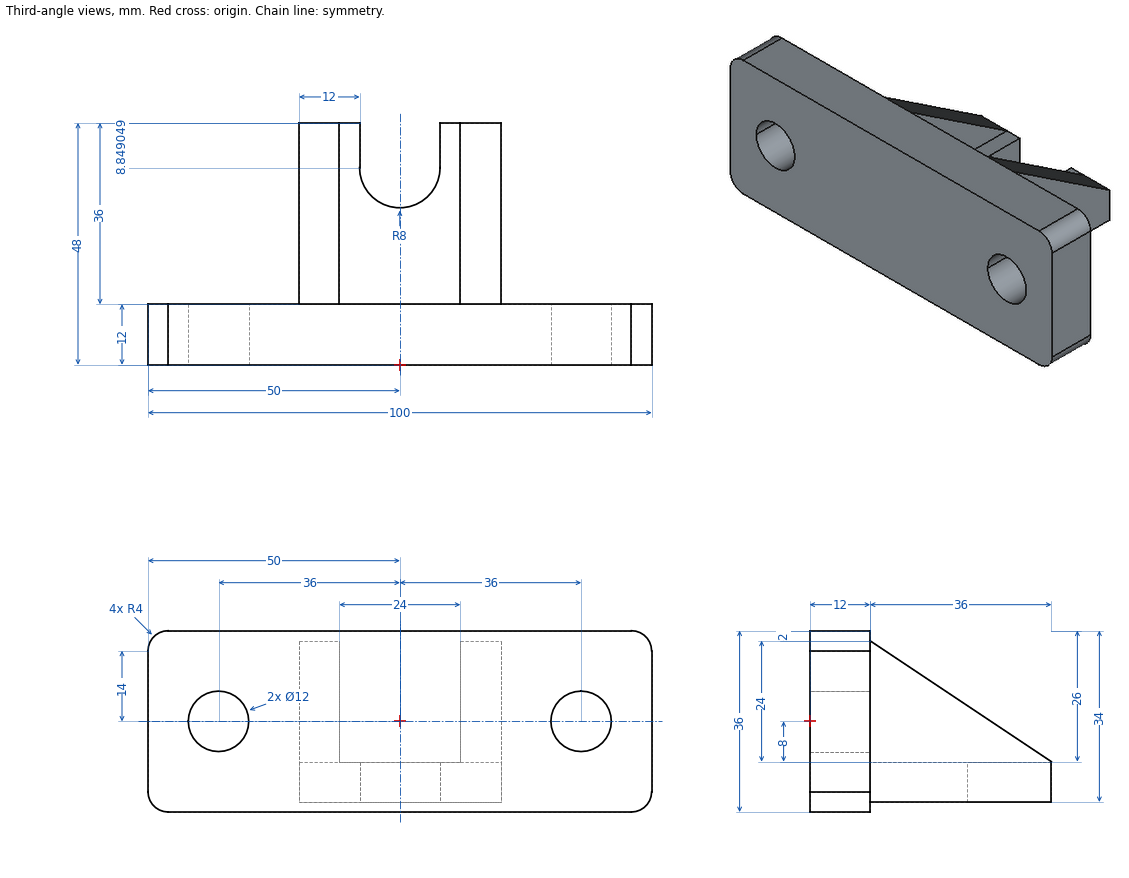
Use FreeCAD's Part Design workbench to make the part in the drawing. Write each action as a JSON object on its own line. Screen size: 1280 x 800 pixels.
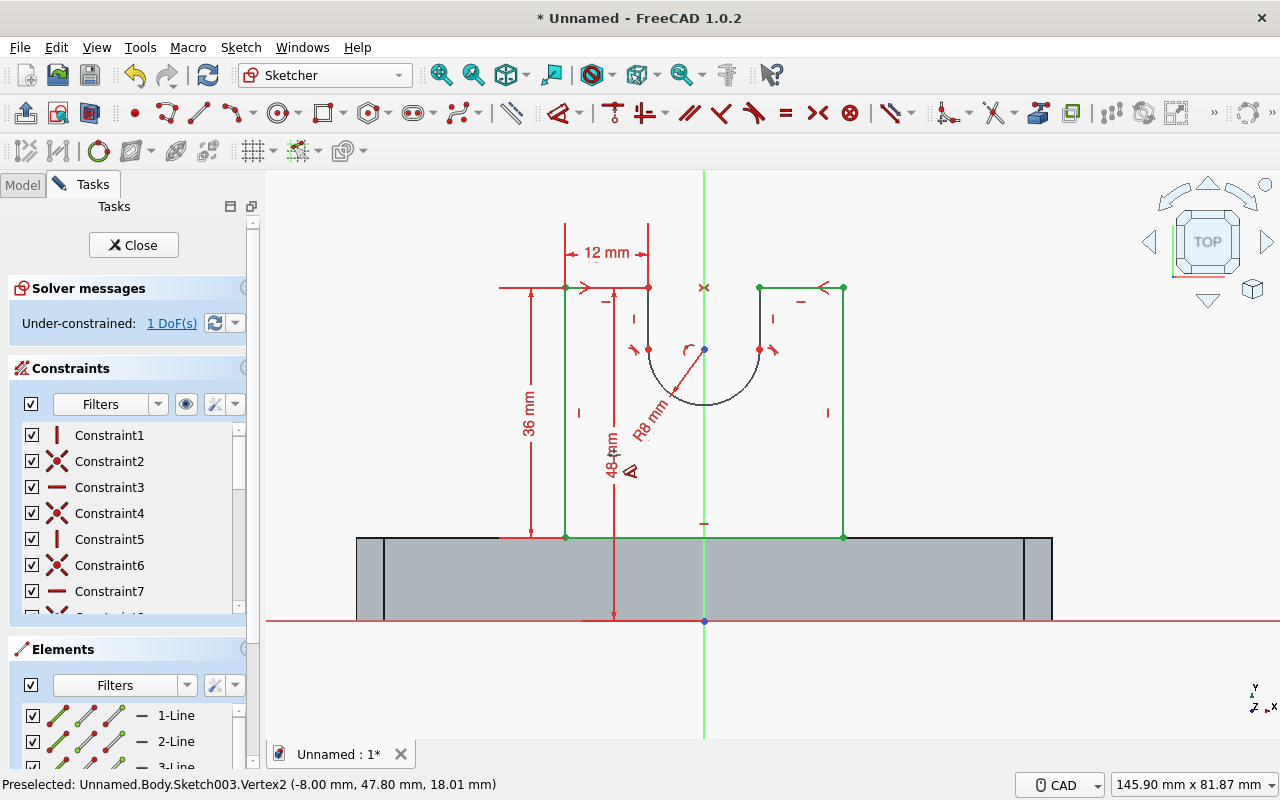
{"action": "left_click", "coordinate": [648, 331]}
{"action": "left_click", "coordinate": [614, 319]}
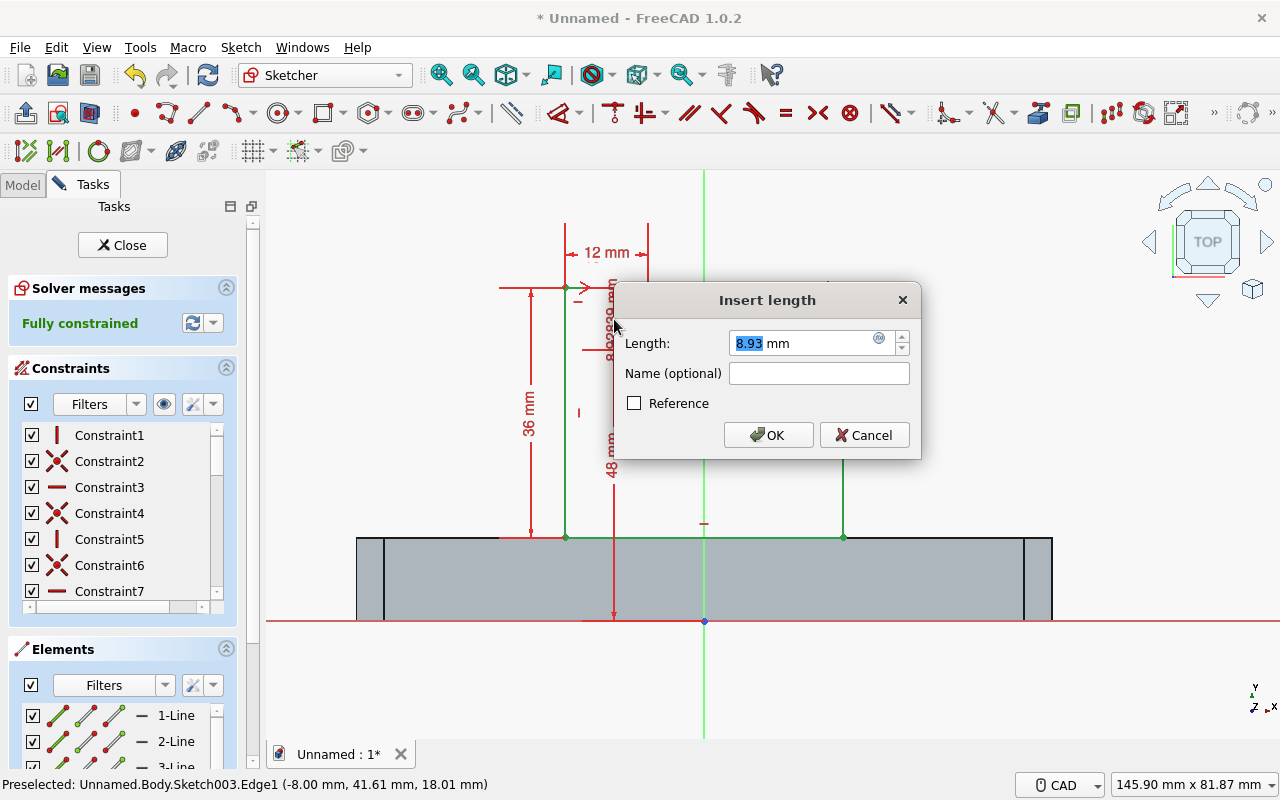
{"action": "type", "text": "8.849049"}
{"action": "key", "text": "Return"}
{"action": "key", "text": "Escape"}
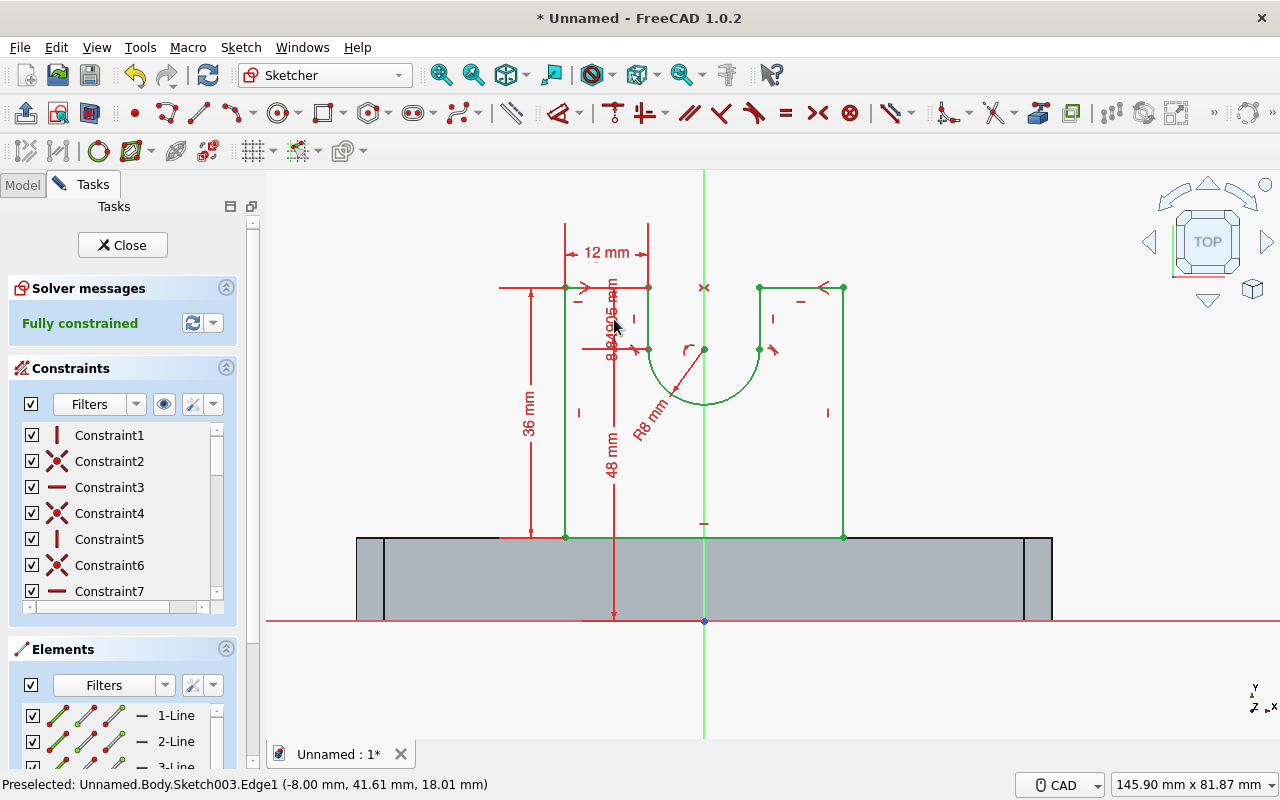
{"action": "left_click", "coordinate": [123, 245]}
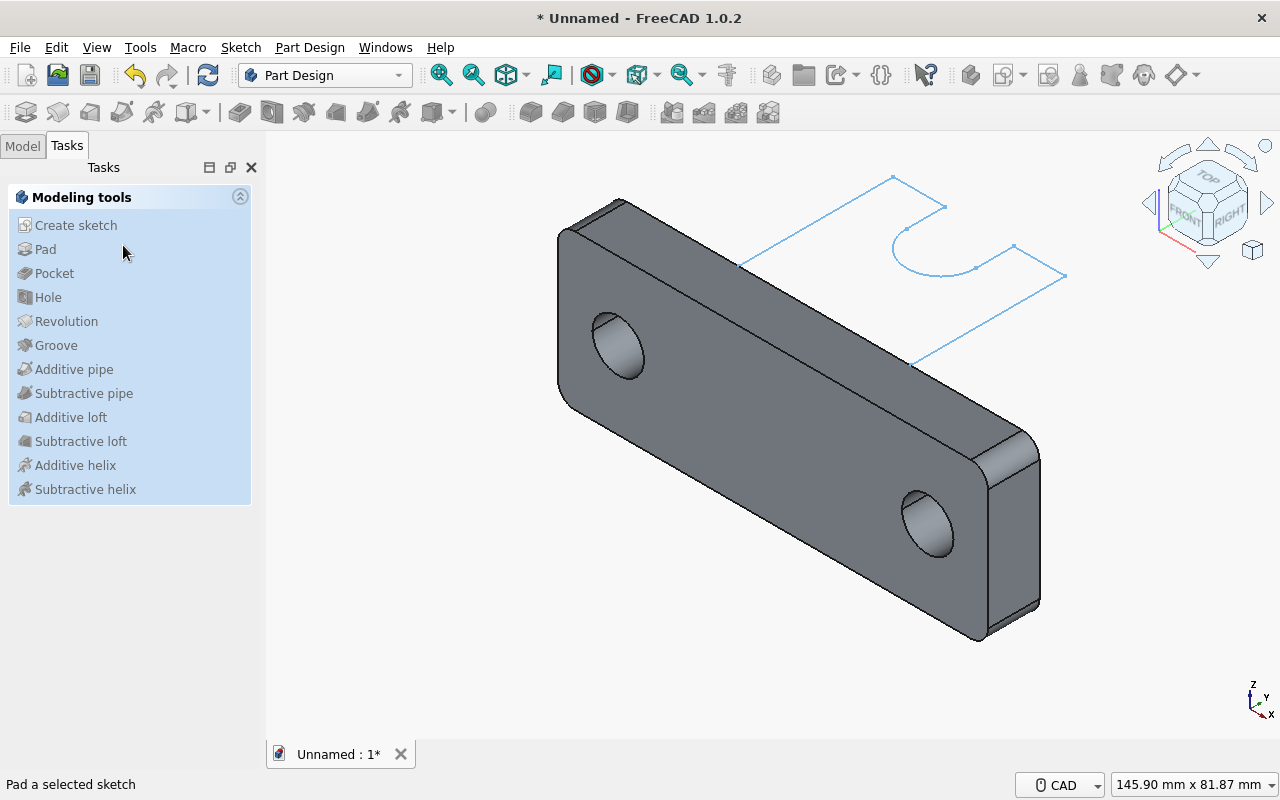
{"action": "left_click", "coordinate": [26, 112]}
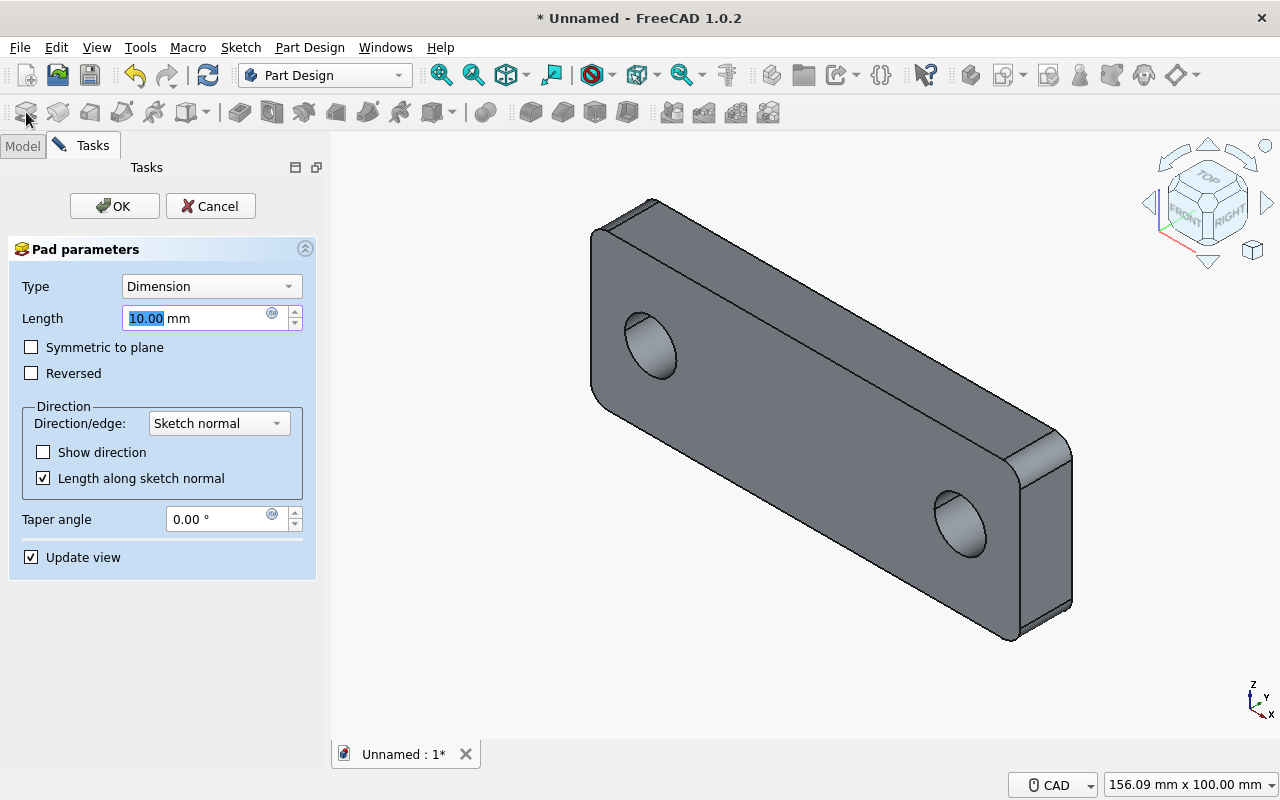
{"action": "type", "text": "34"}
{"action": "key", "text": "Tab"}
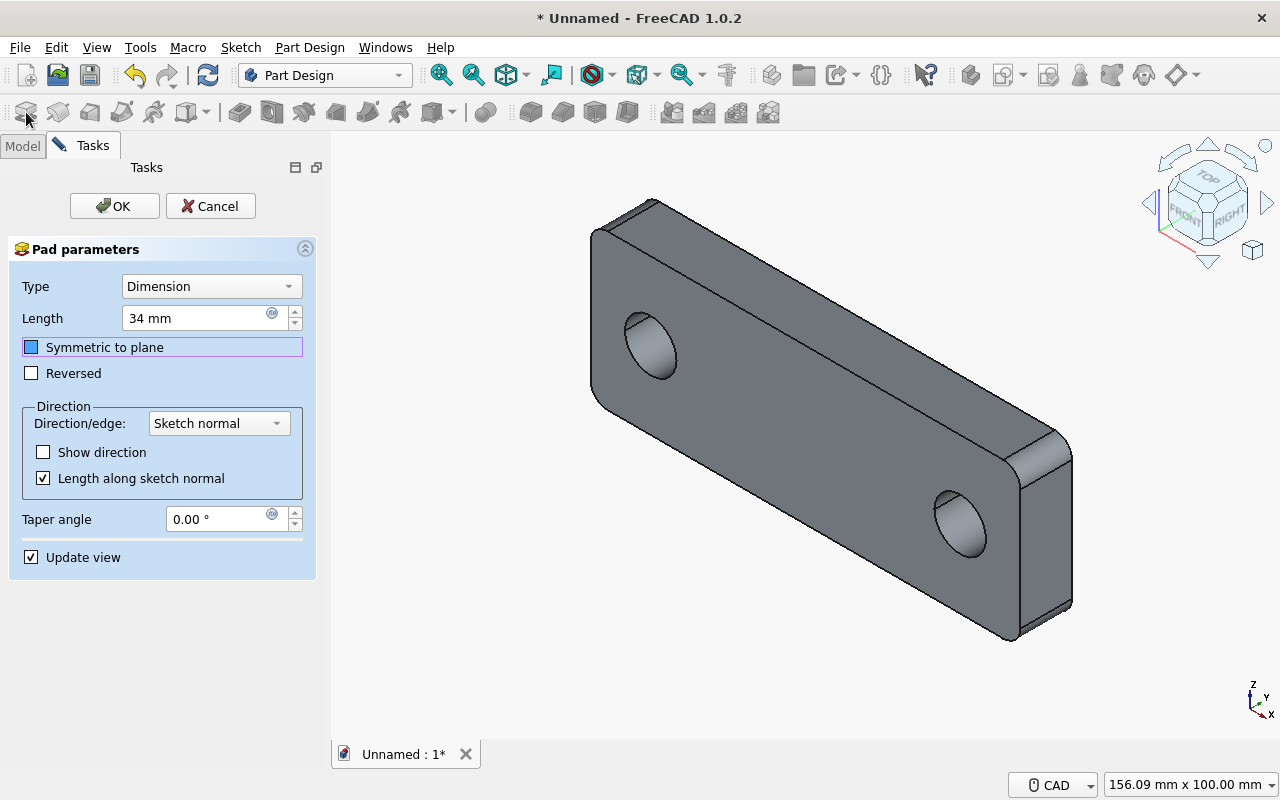
{"action": "left_click", "coordinate": [30, 373]}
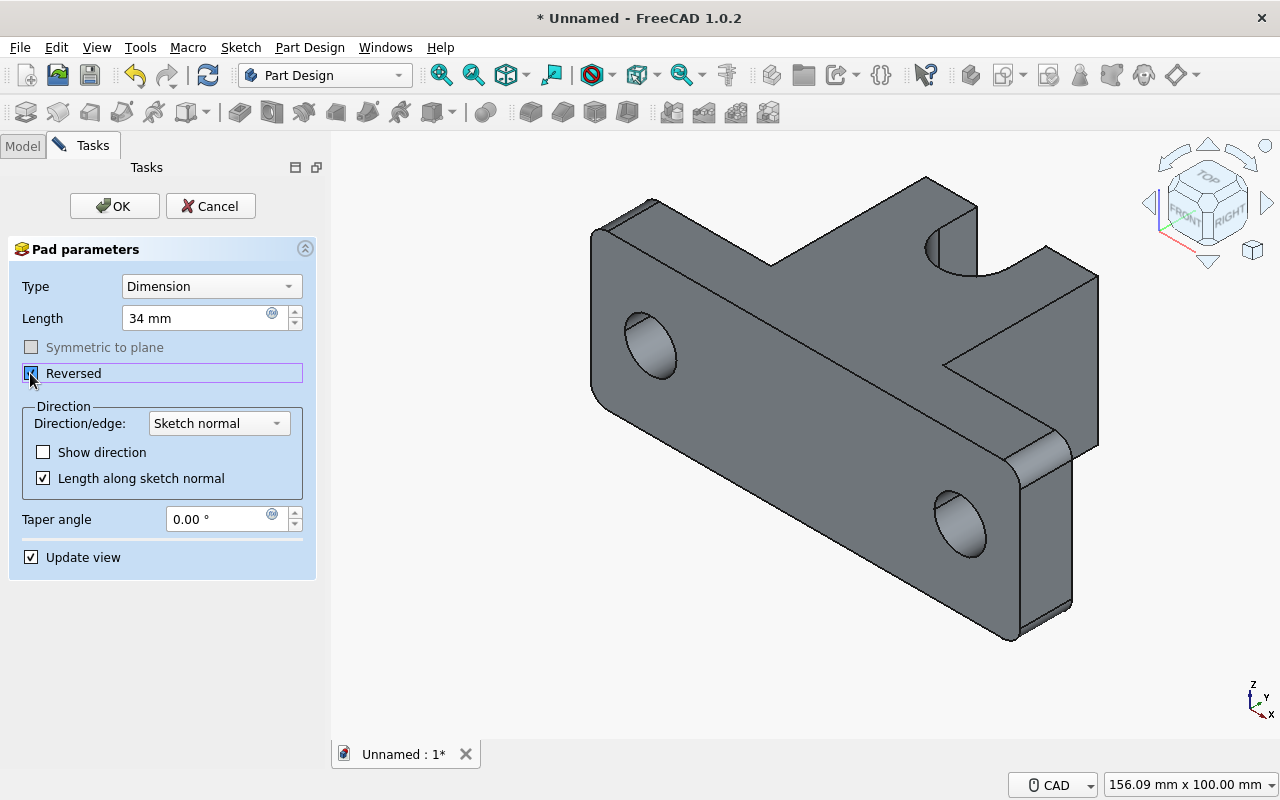
{"action": "left_click", "coordinate": [115, 206]}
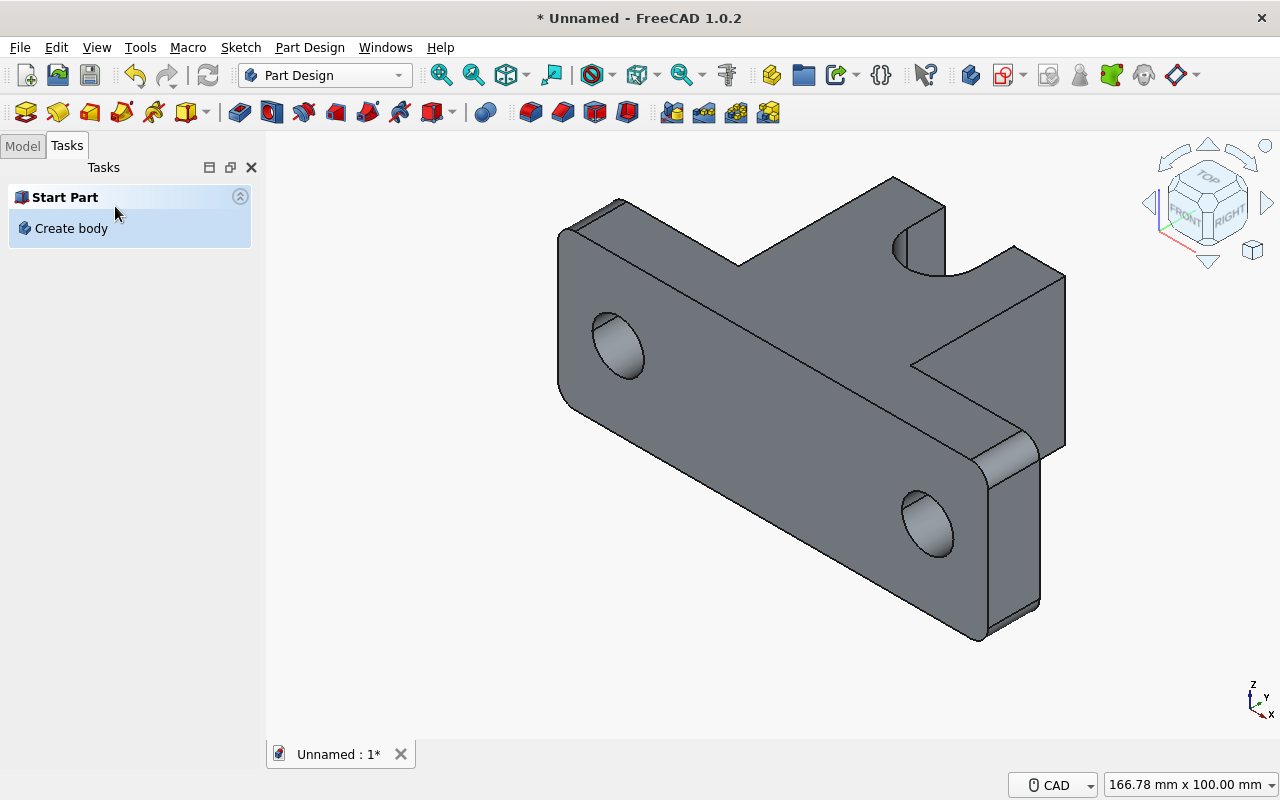
{"action": "left_click", "coordinate": [442, 76]}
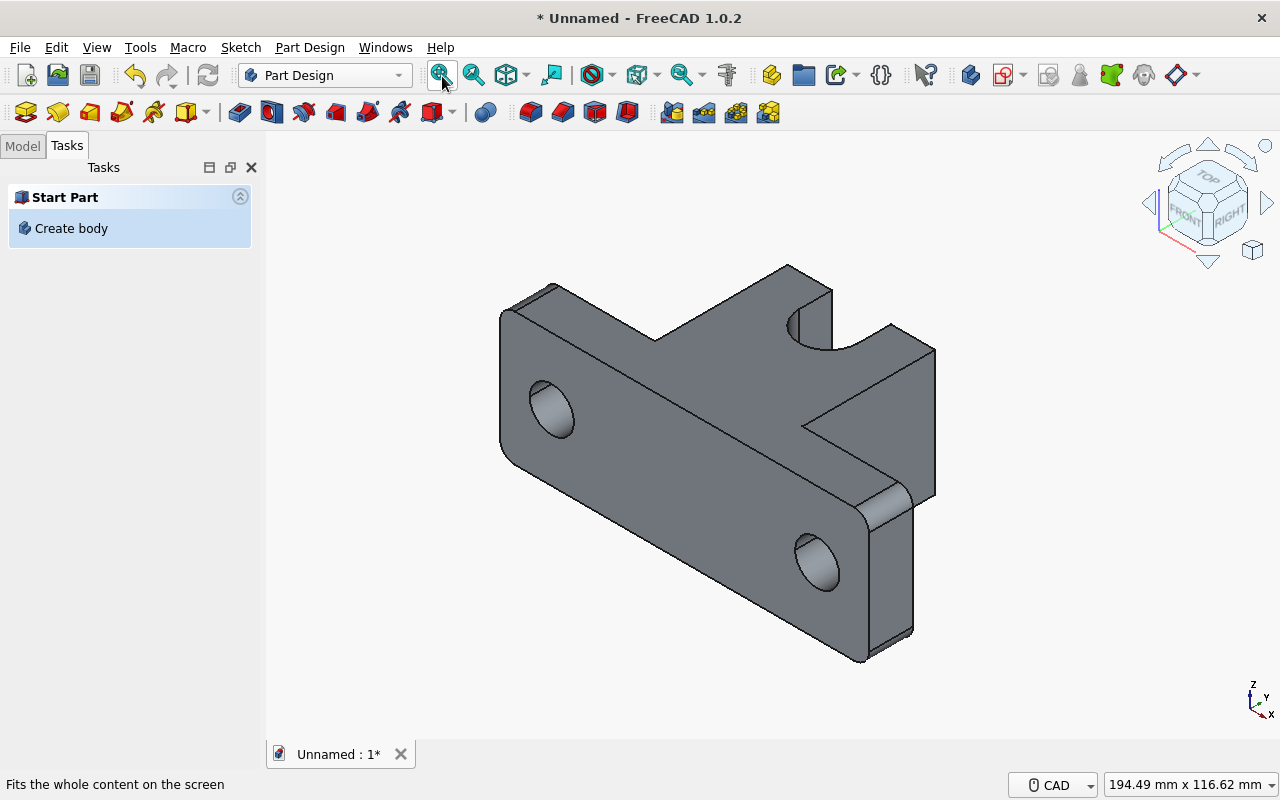
{"action": "key", "text": "6"}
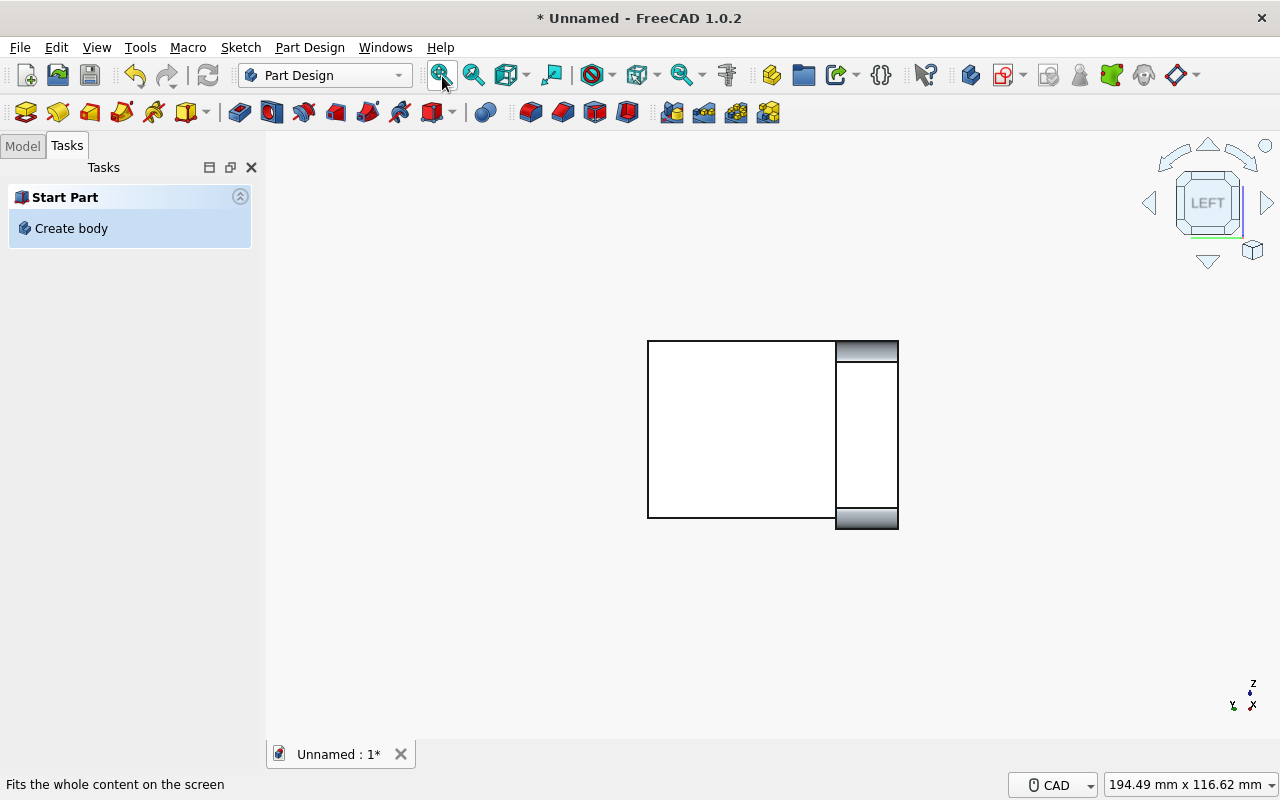
{"action": "left_click", "coordinate": [442, 76]}